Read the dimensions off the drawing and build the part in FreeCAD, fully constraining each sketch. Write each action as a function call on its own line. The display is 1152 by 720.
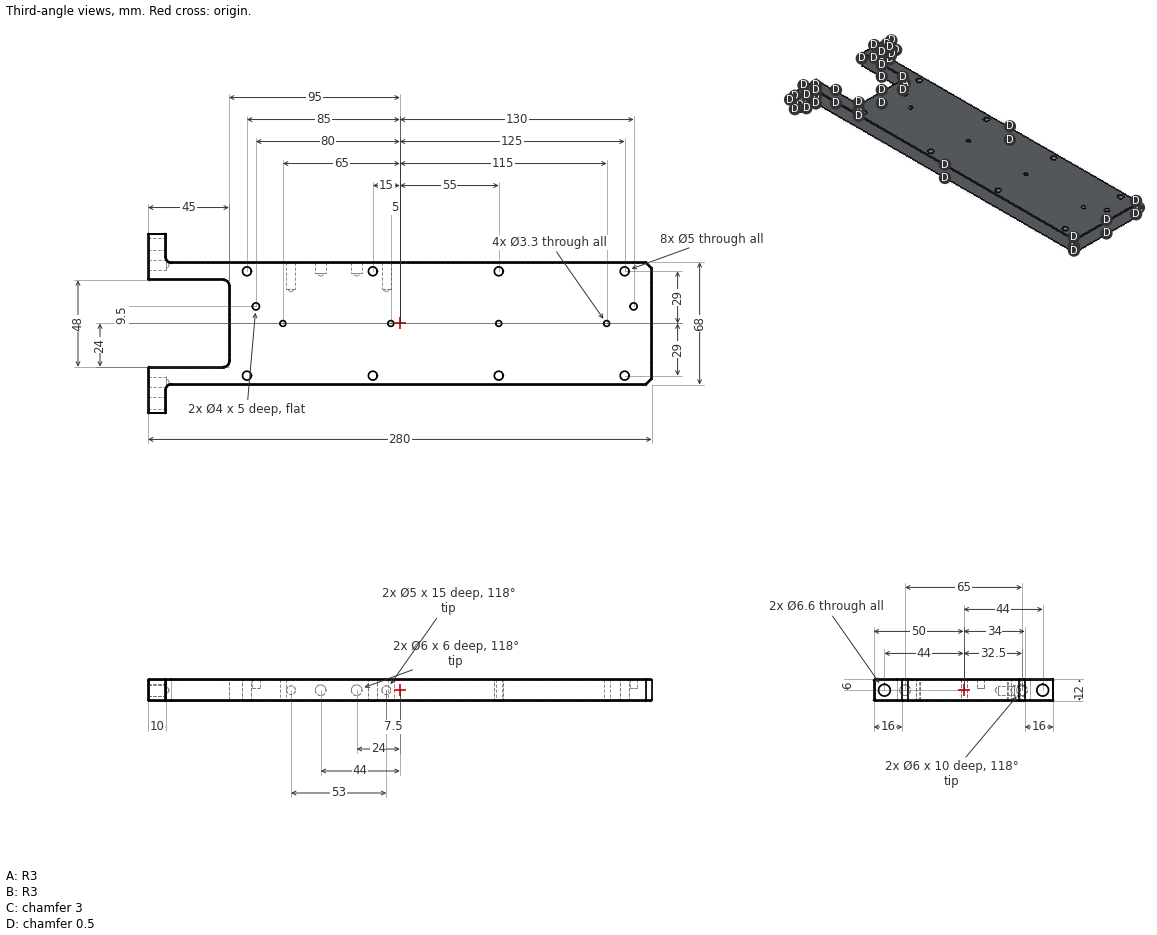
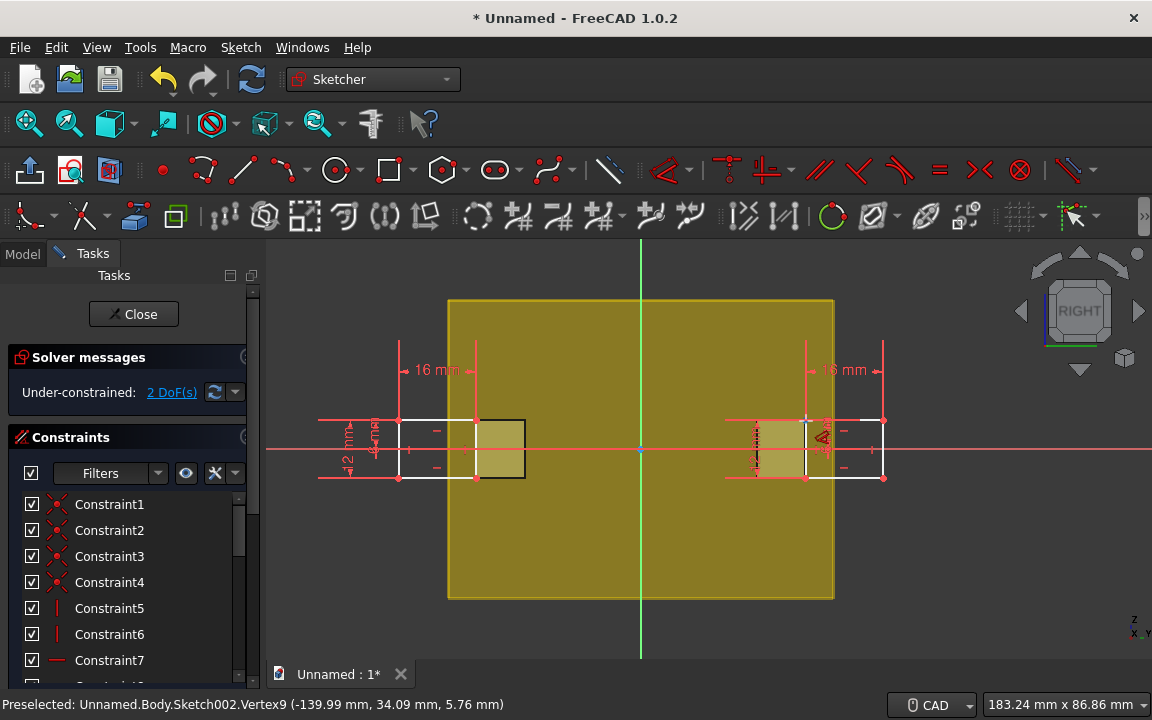
click(399, 420)
click(520, 386)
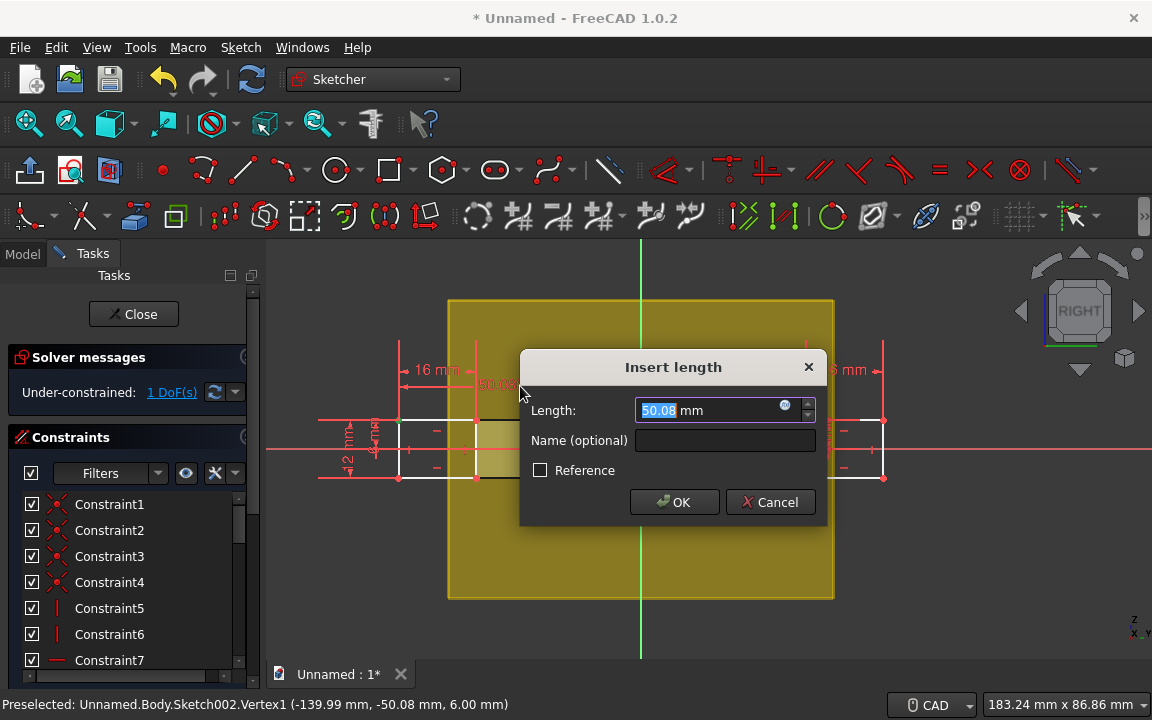
text(50)
key(Return)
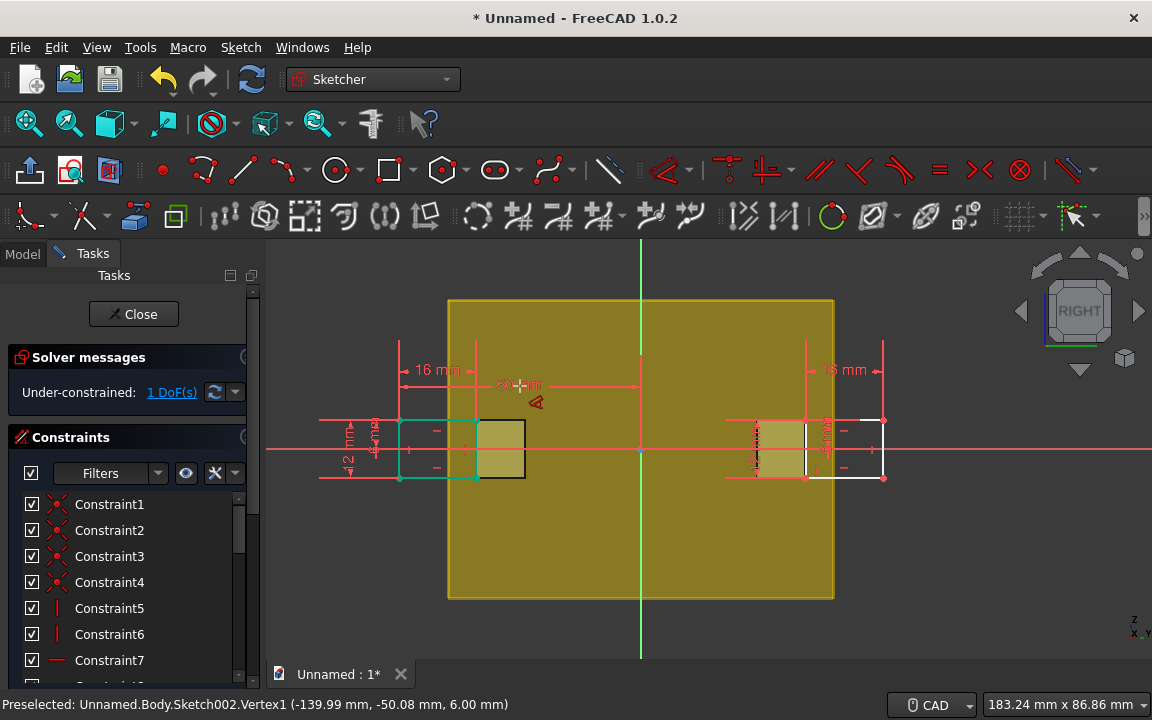
click(806, 420)
click(723, 386)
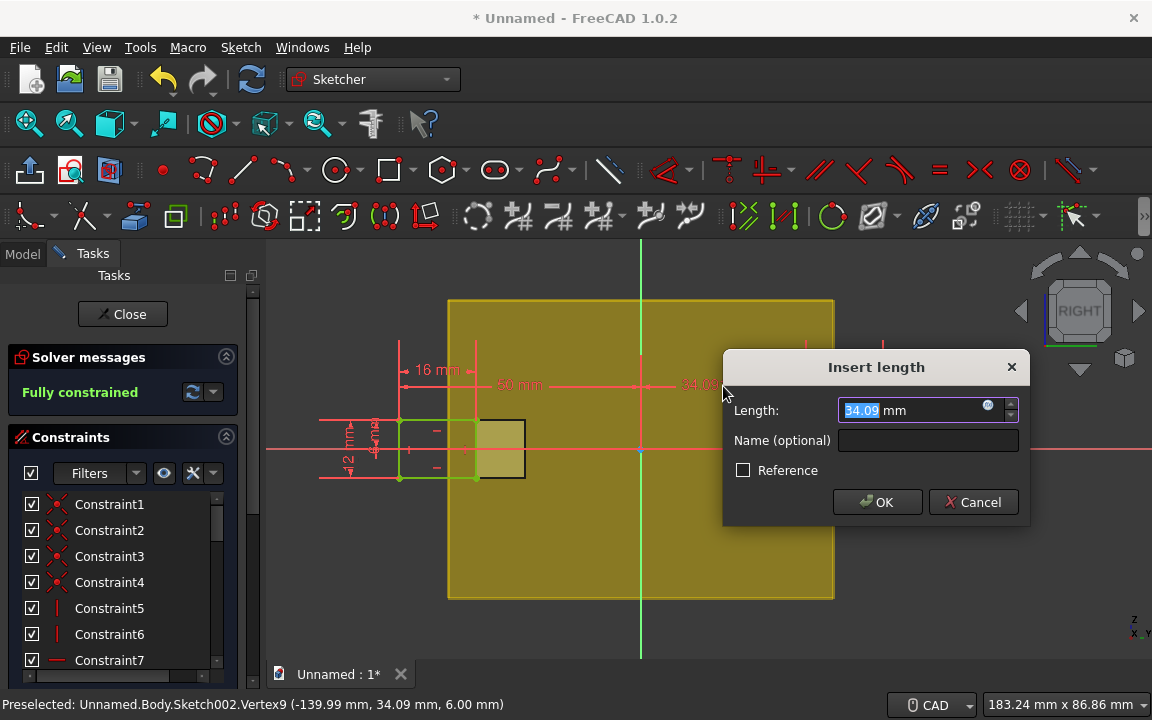
text(34)
key(Return)
key(Escape)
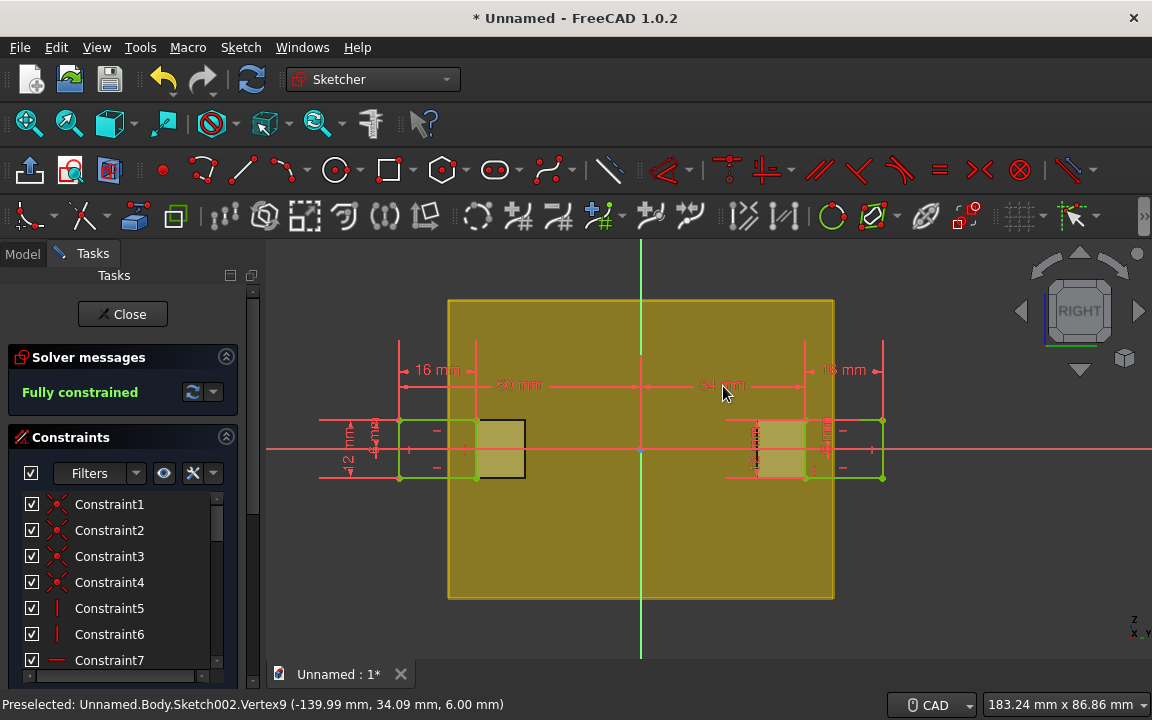
click(123, 314)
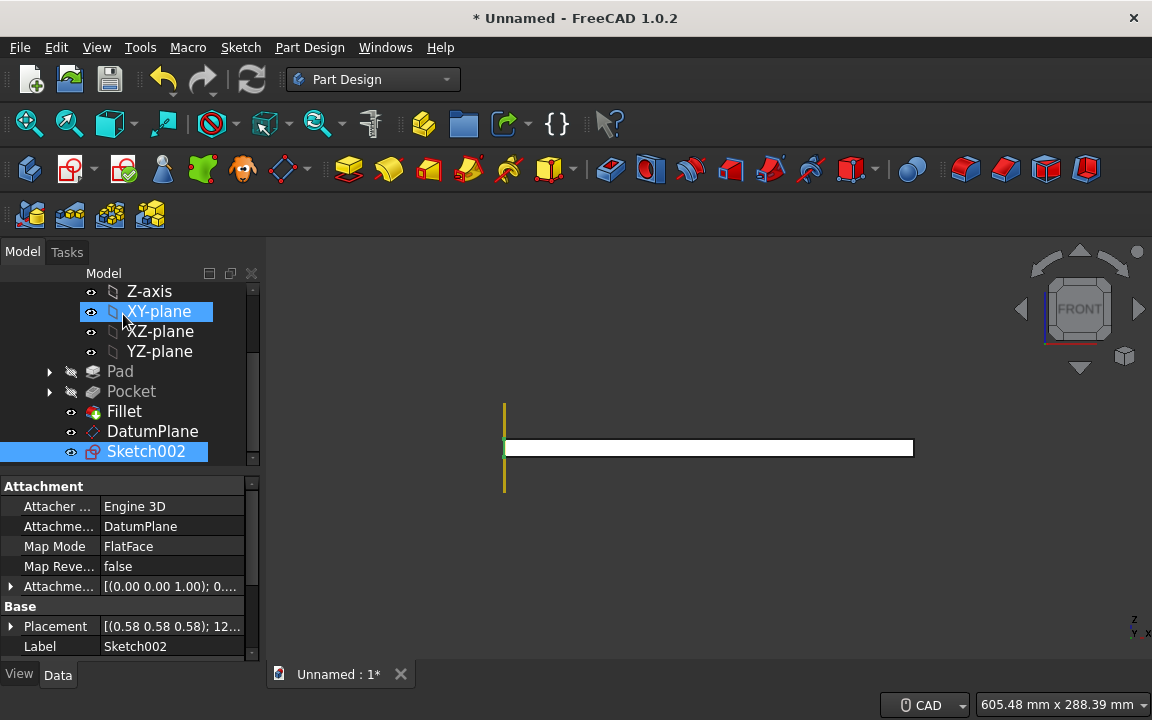
click(350, 170)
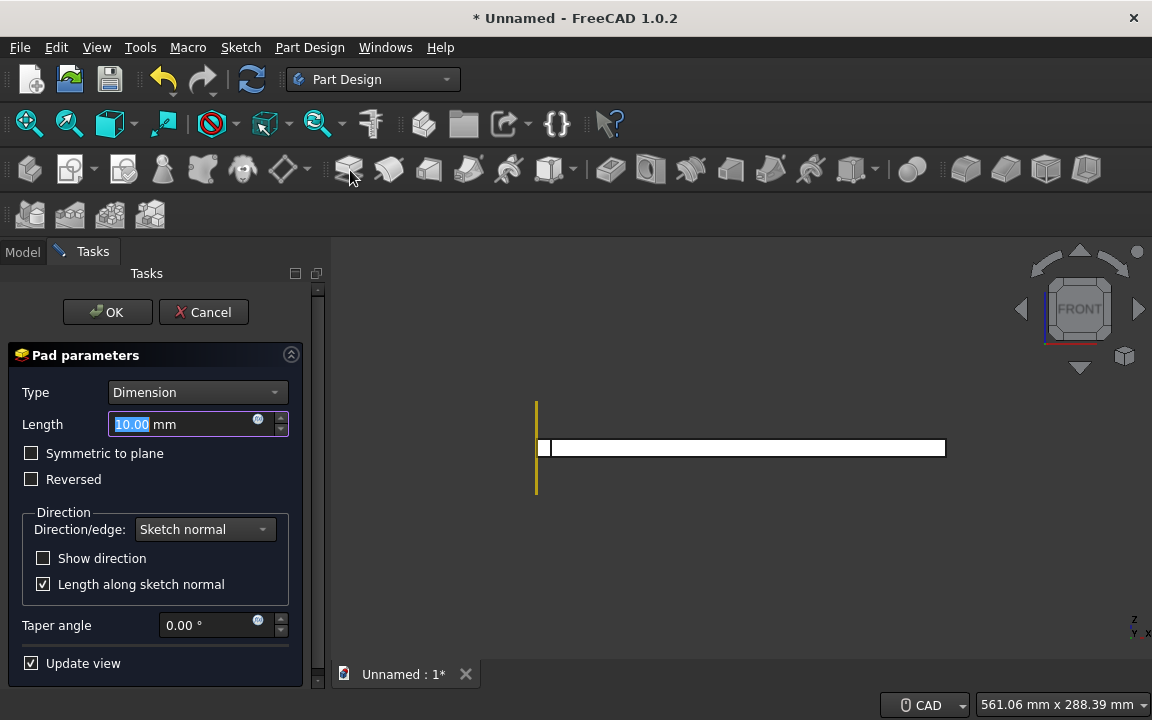
text(10)
key(Tab)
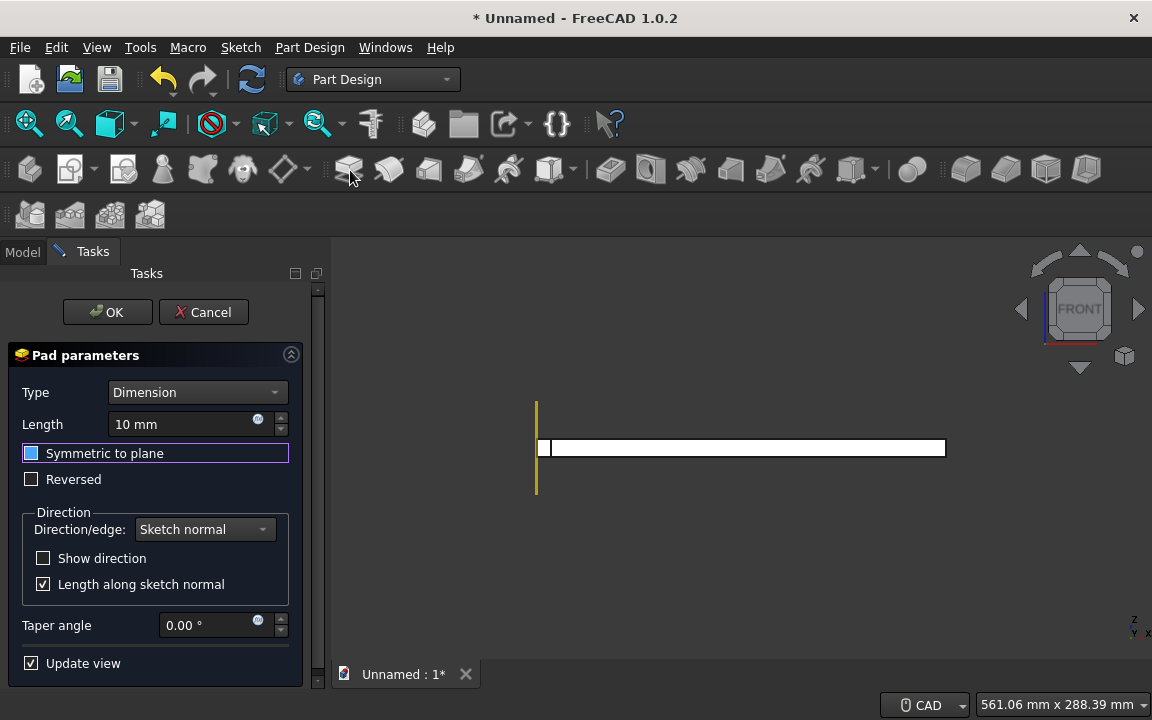
click(108, 312)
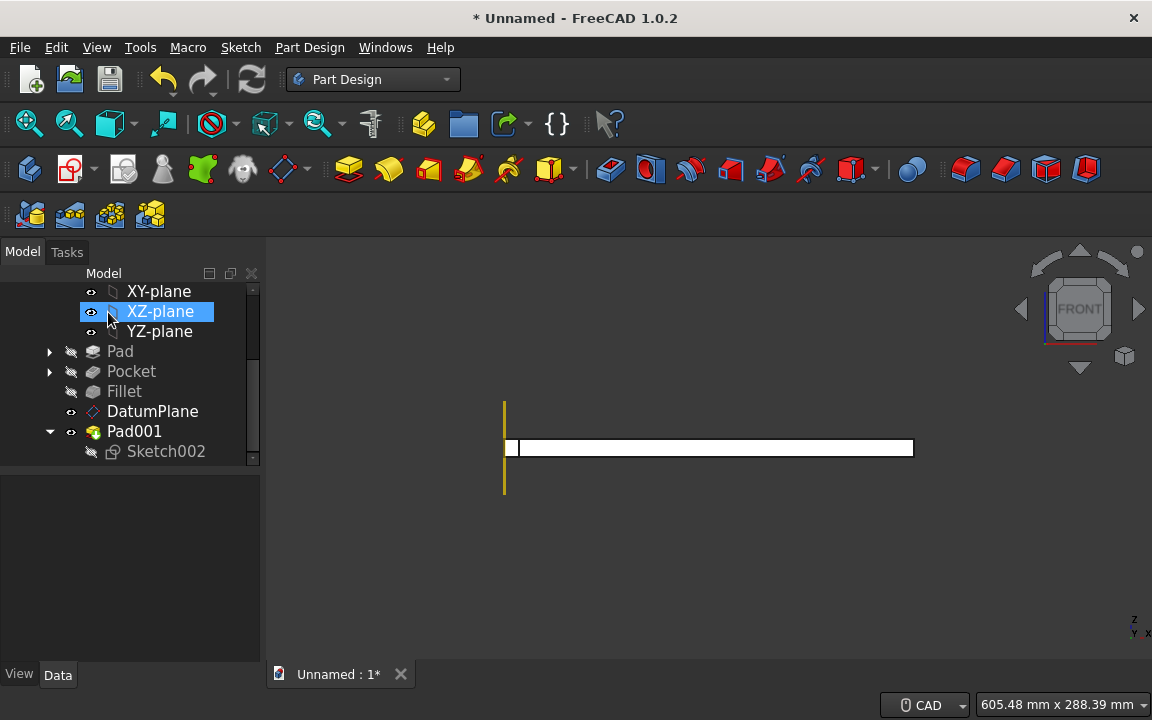
click(116, 412)
key(space)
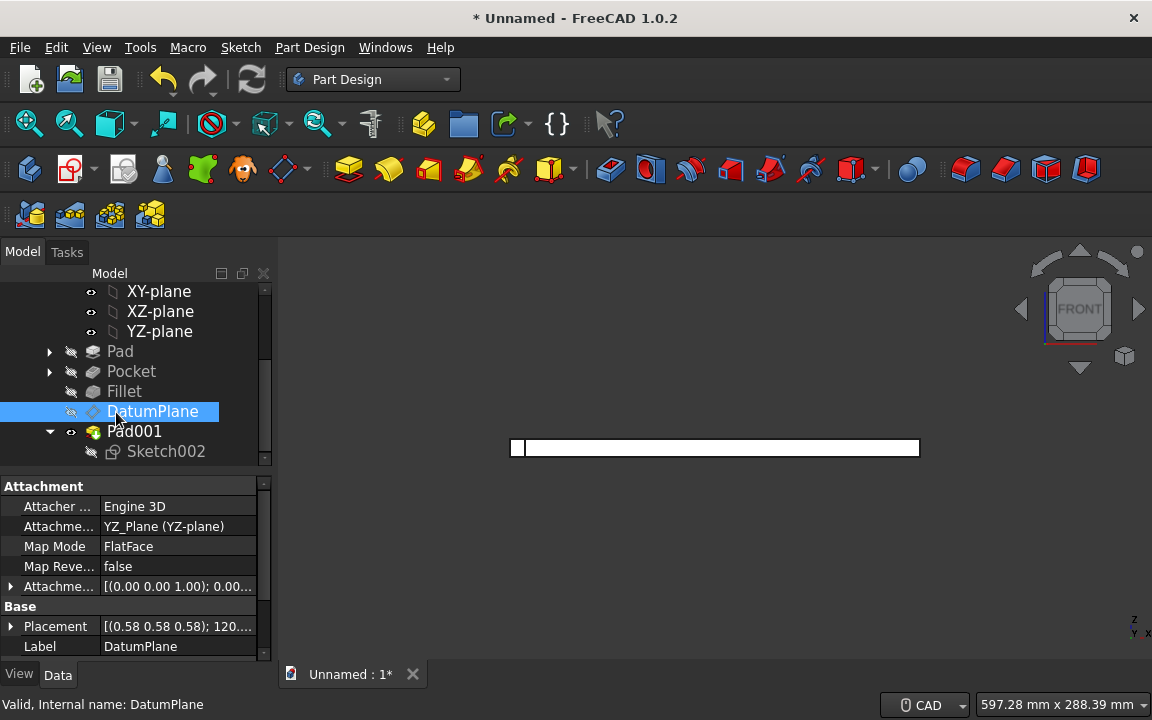
scroll(525, 447, up, 5)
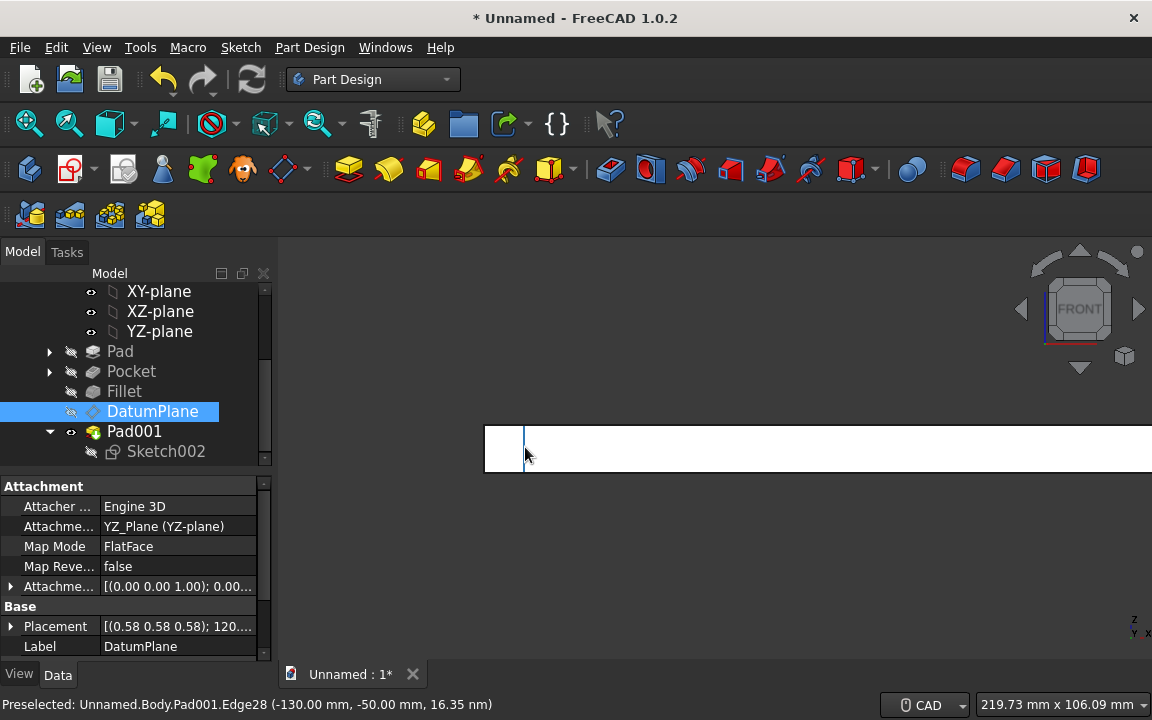
key(v)
key(f)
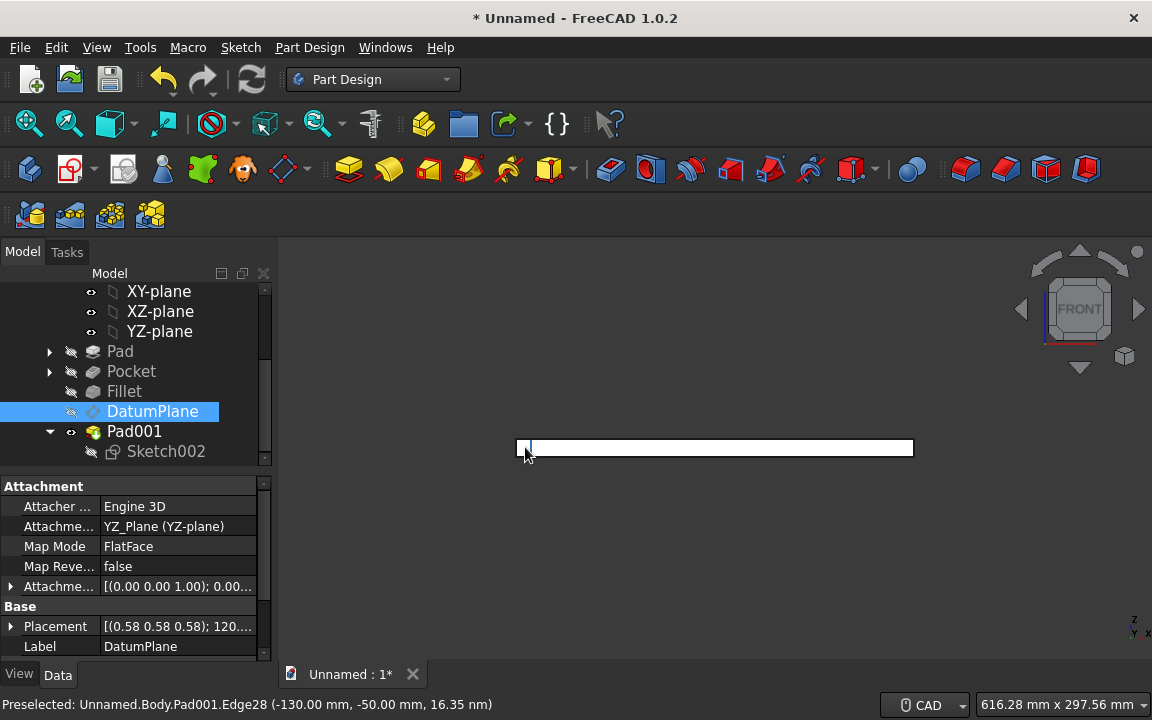
key(0)